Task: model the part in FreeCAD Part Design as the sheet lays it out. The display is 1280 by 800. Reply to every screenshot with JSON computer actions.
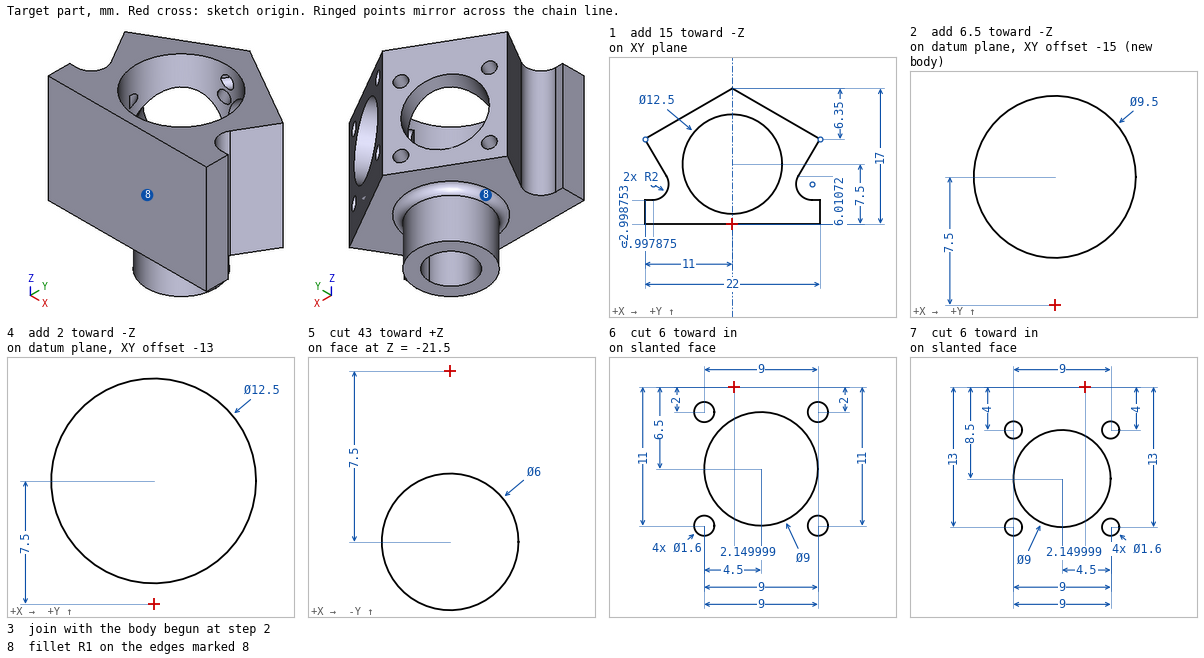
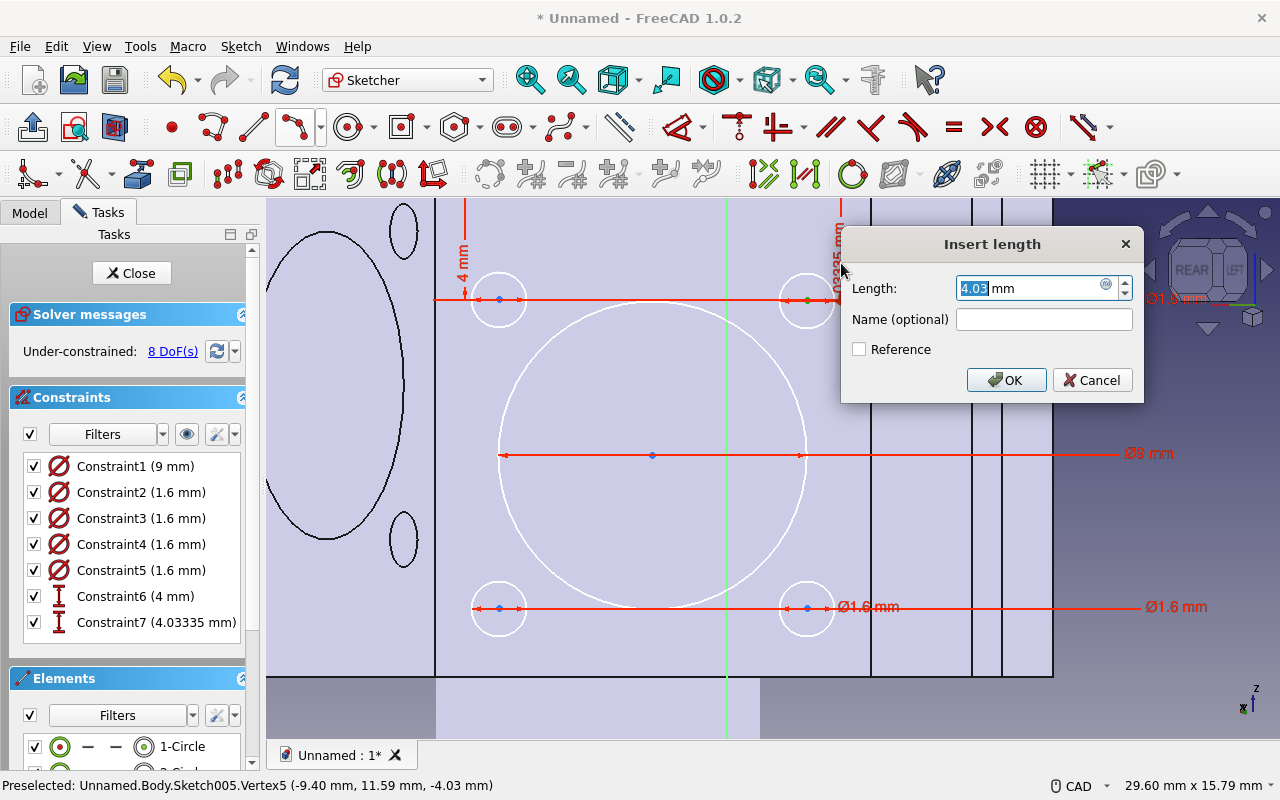
{"action": "type", "text": "4"}
{"action": "key", "text": "Return"}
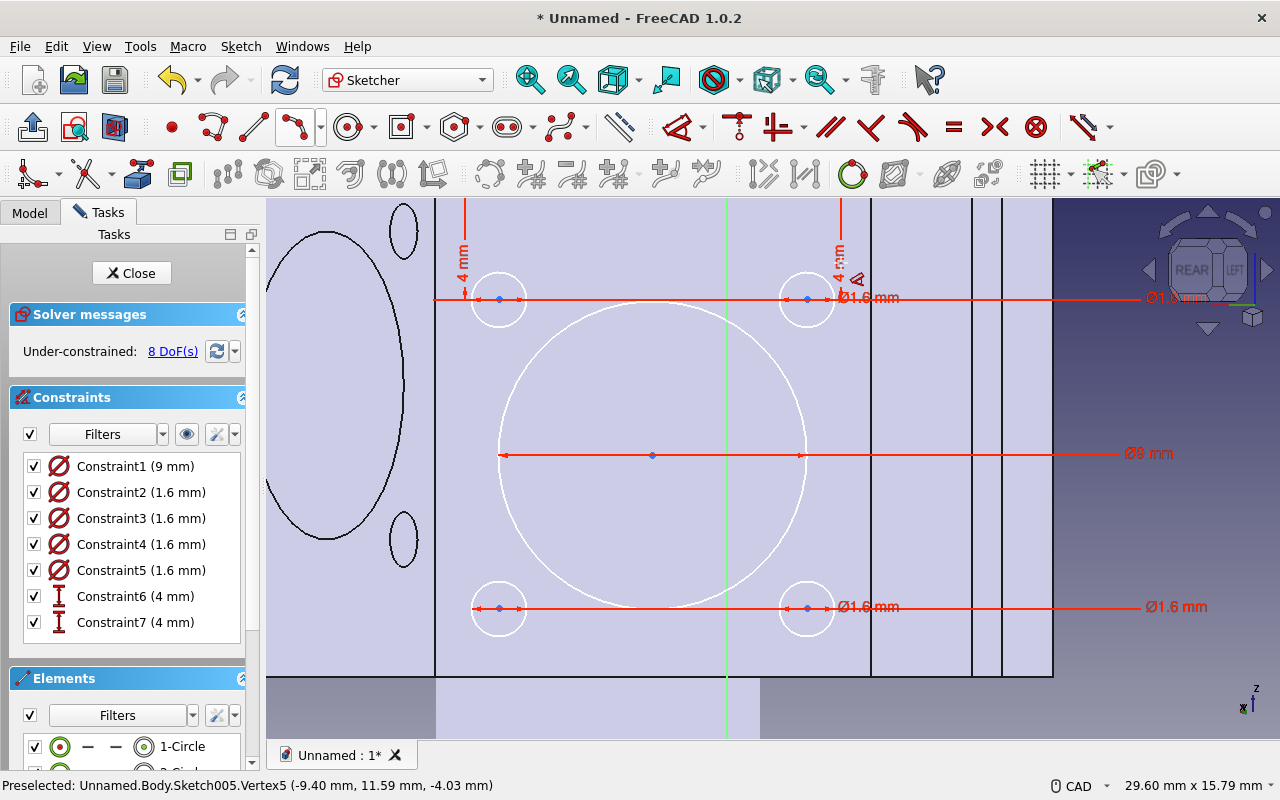
{"action": "left_click", "coordinate": [807, 609]}
{"action": "left_click", "coordinate": [841, 417]}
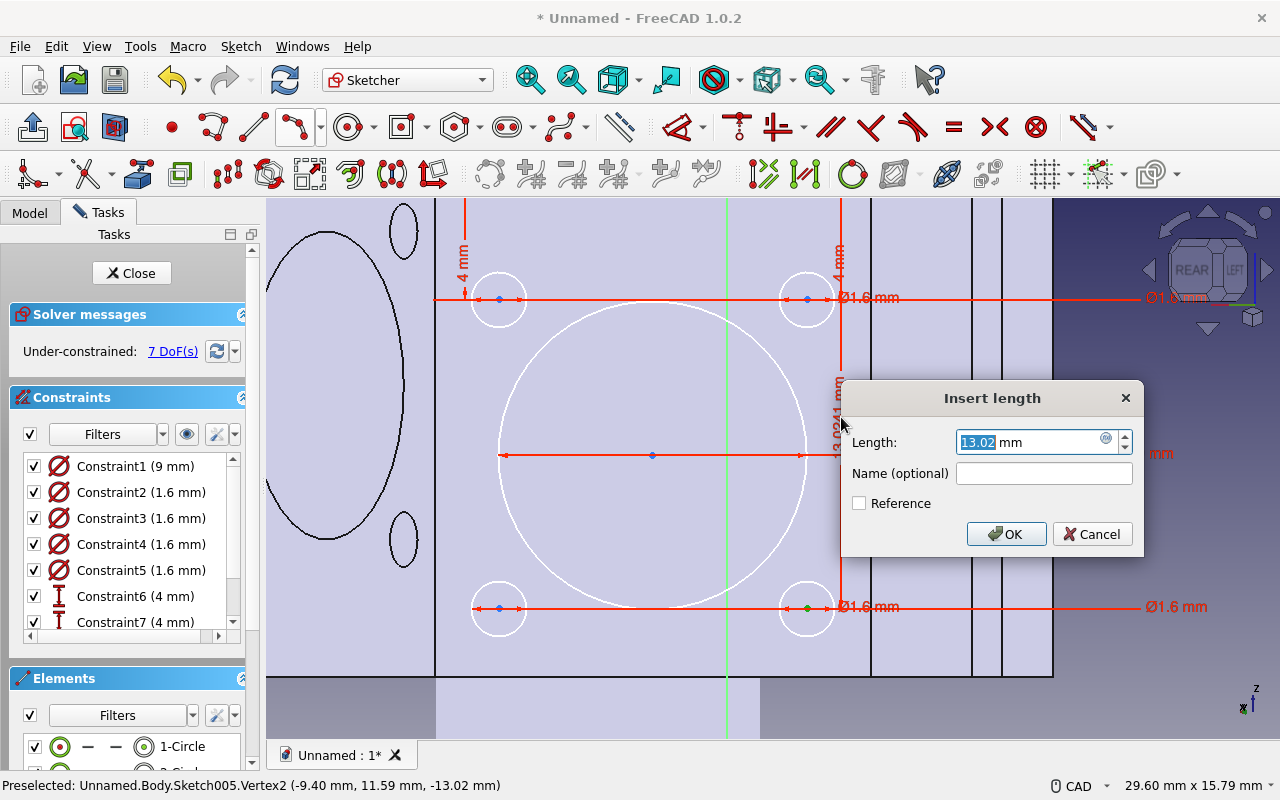
{"action": "type", "text": "13"}
{"action": "key", "text": "Return"}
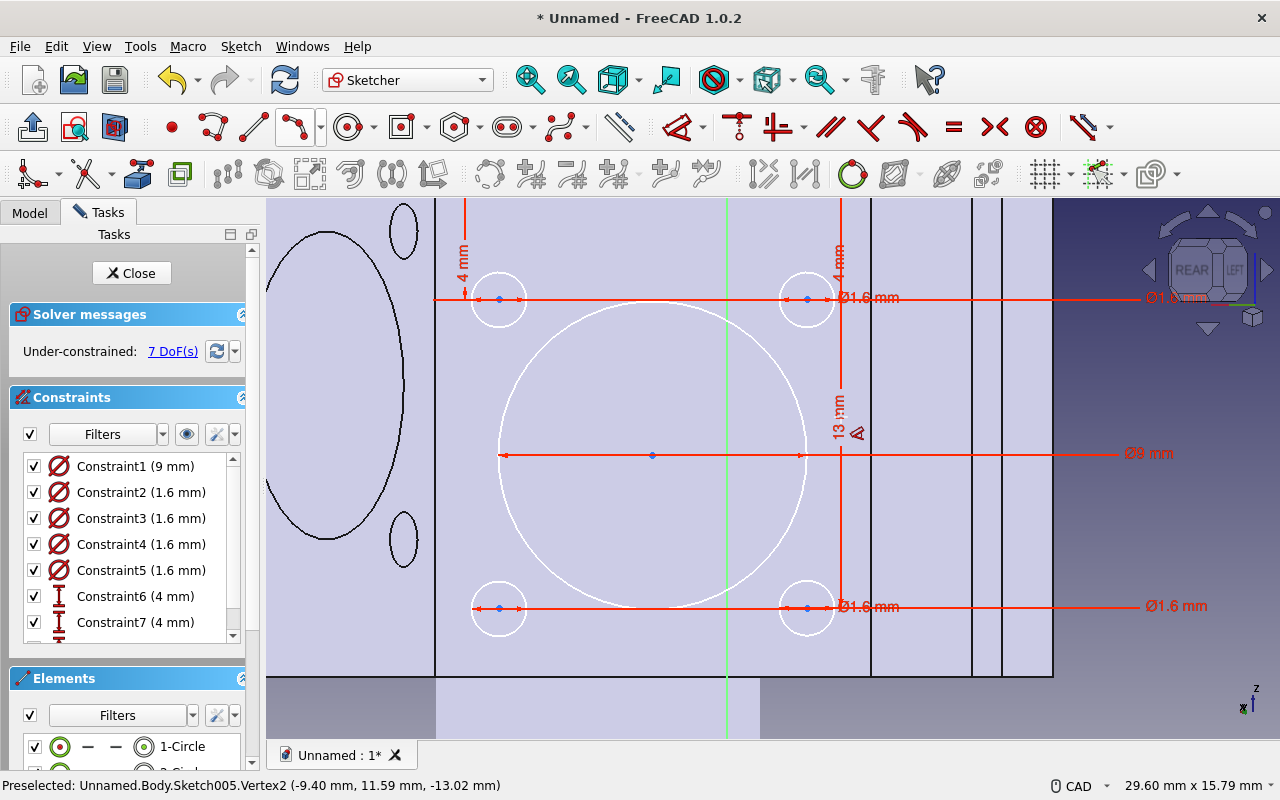
{"action": "left_click", "coordinate": [499, 609]}
{"action": "left_click", "coordinate": [465, 417]}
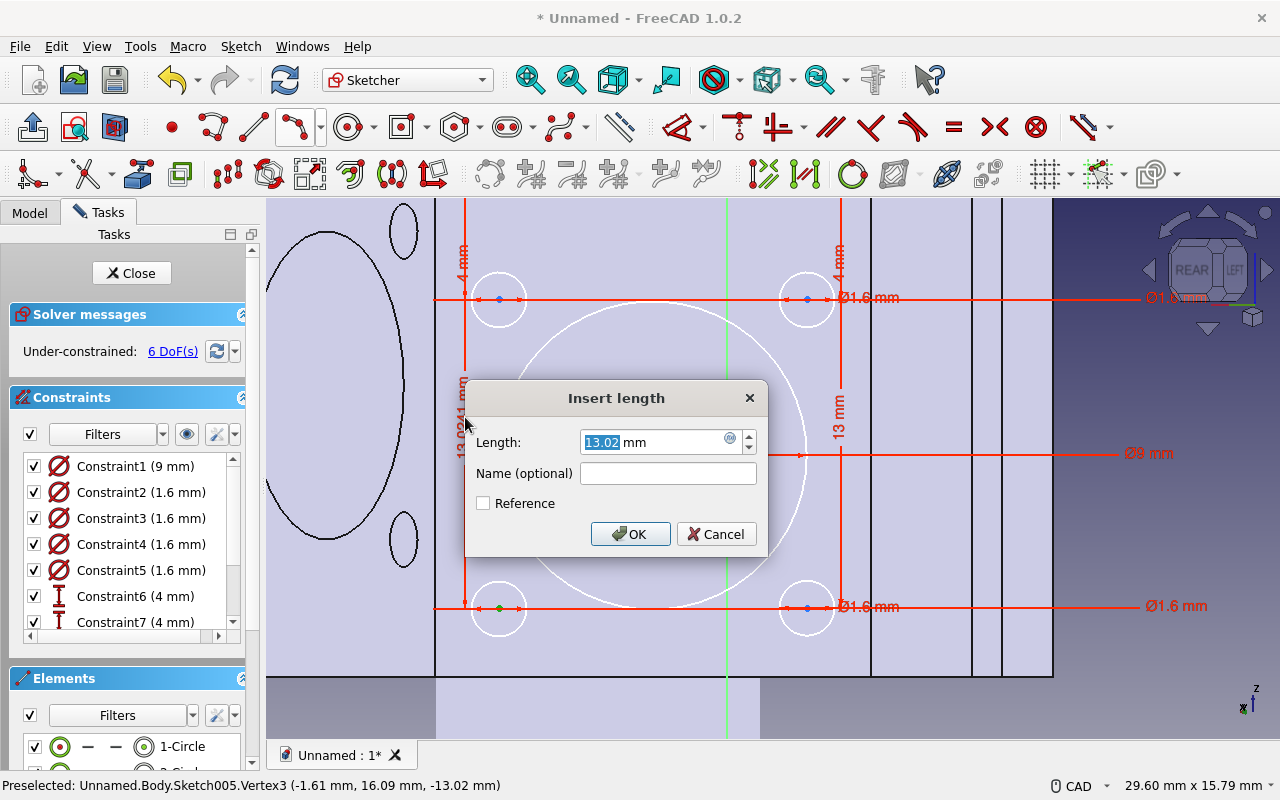
{"action": "type", "text": "13"}
{"action": "key", "text": "Return"}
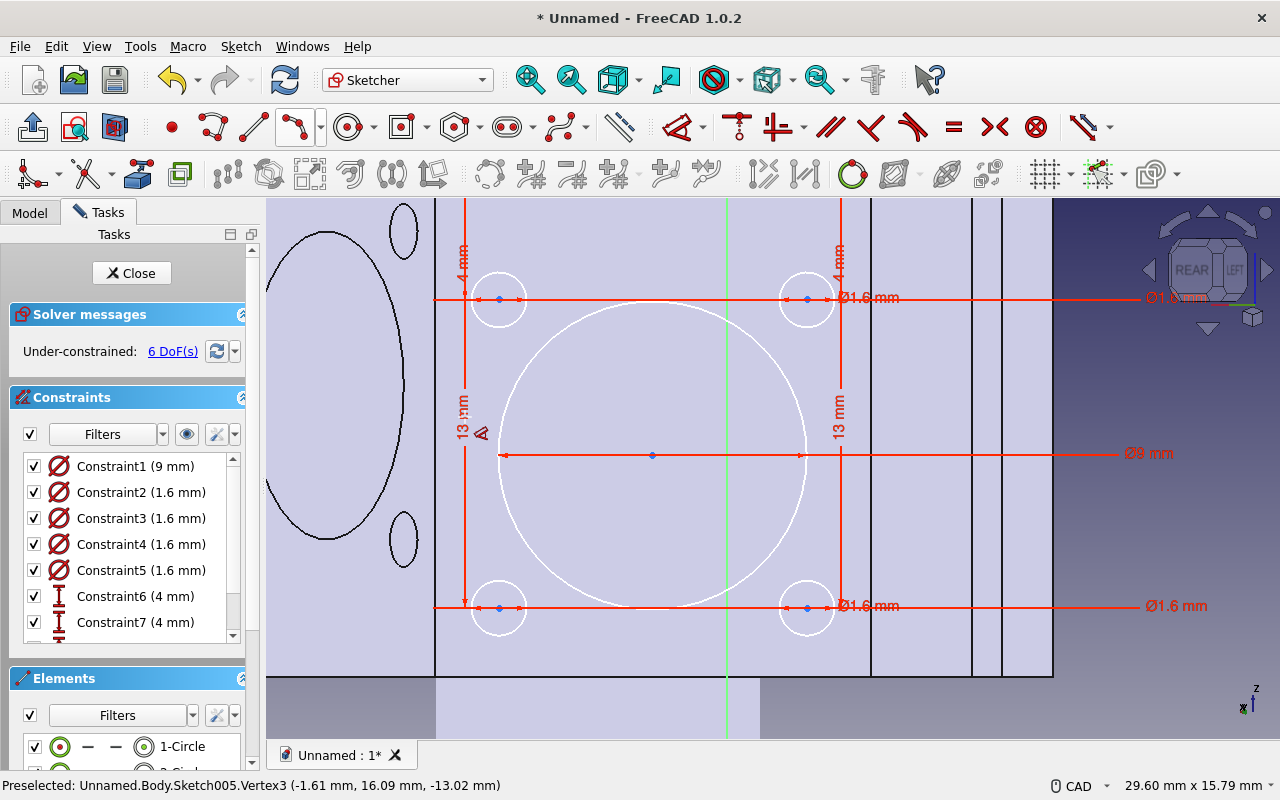
{"action": "left_click", "coordinate": [807, 608]}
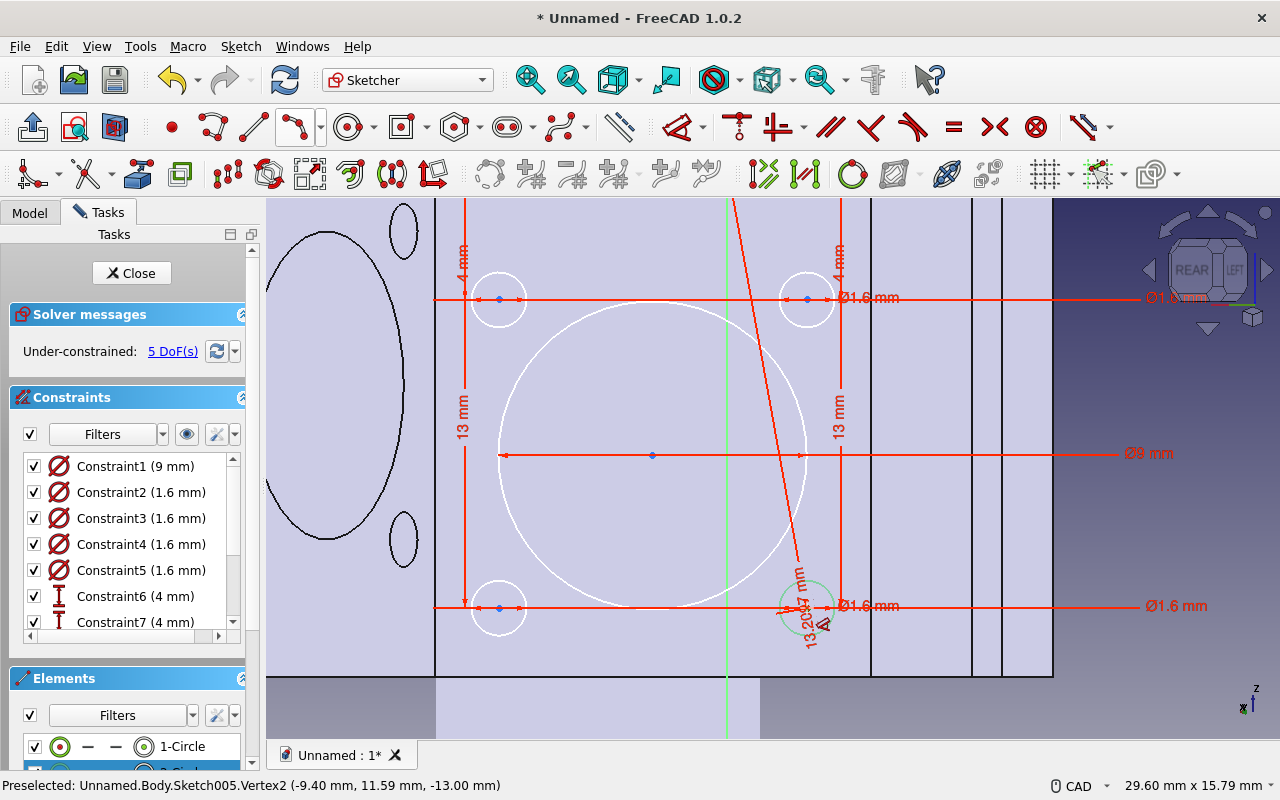
{"action": "left_click", "coordinate": [499, 608]}
{"action": "left_click", "coordinate": [653, 642]}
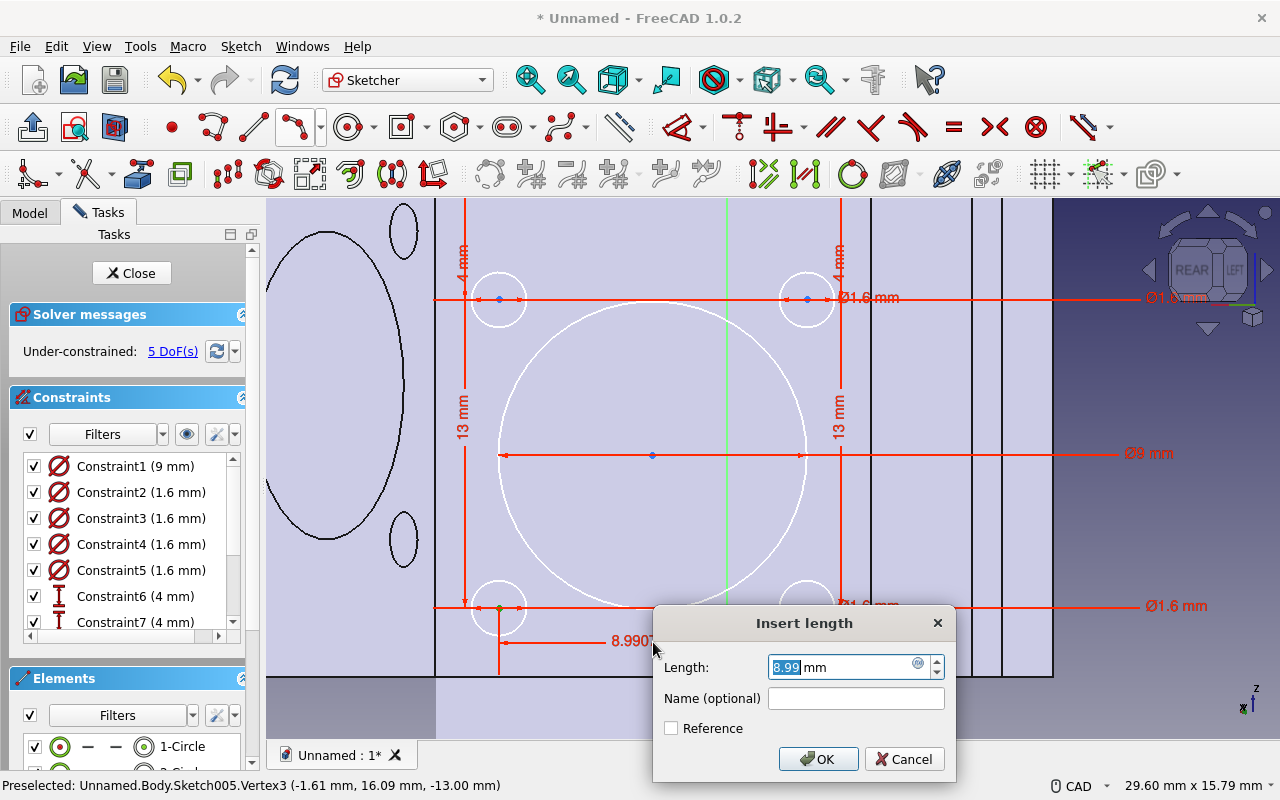
{"action": "type", "text": "9"}
{"action": "key", "text": "Return"}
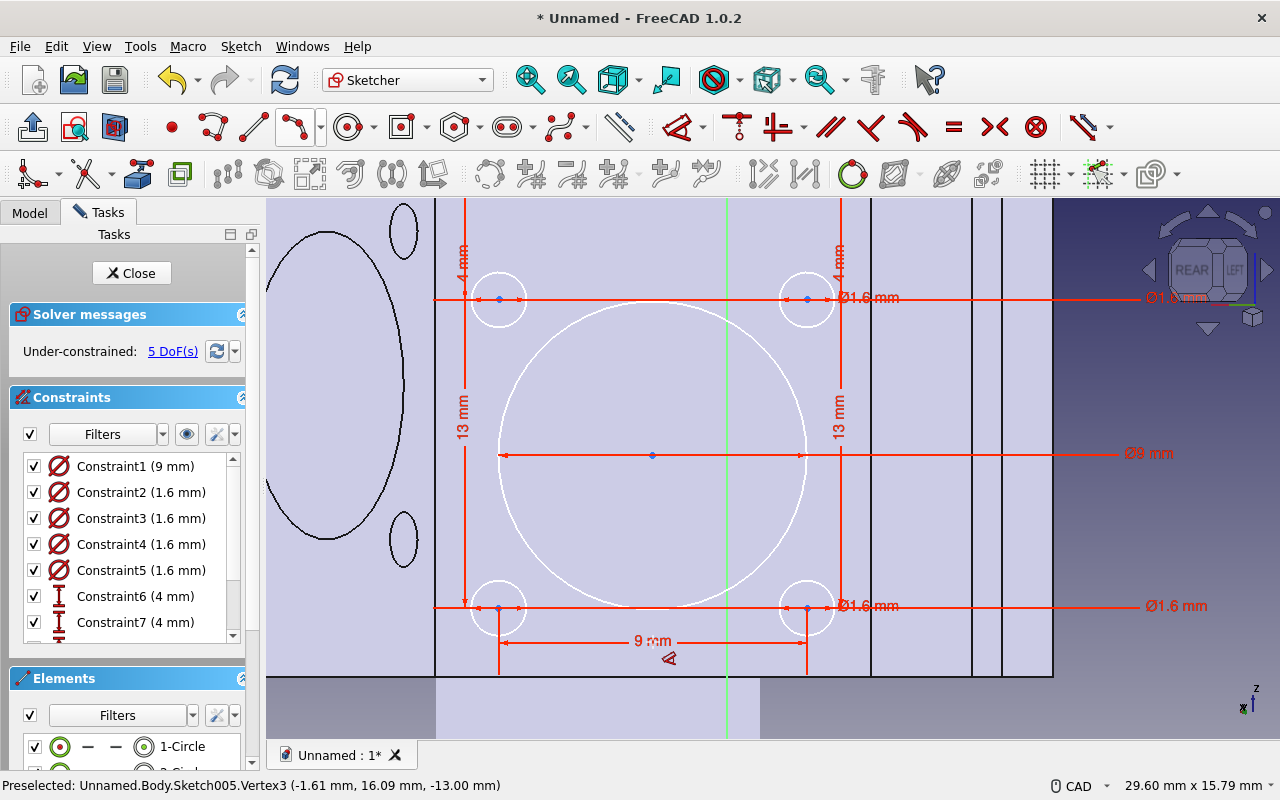
{"action": "left_click", "coordinate": [807, 608]}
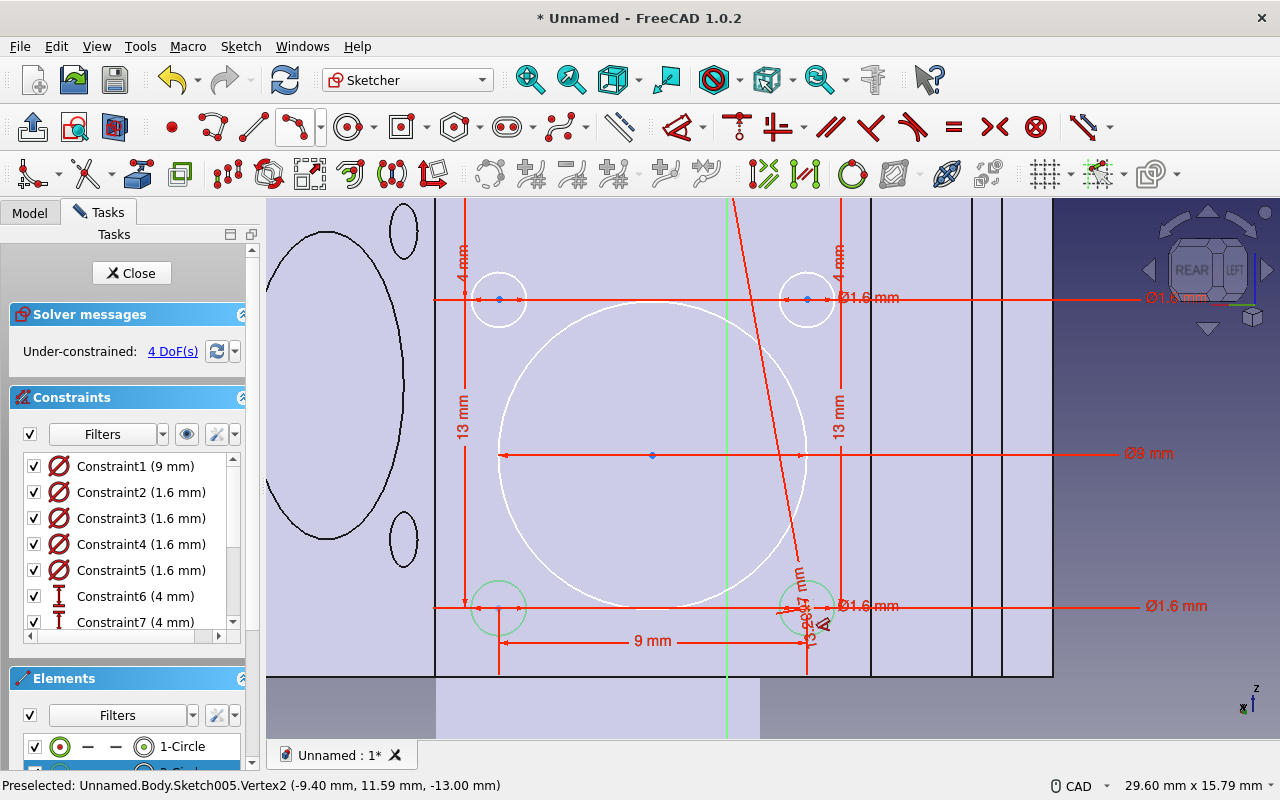
{"action": "left_click", "coordinate": [499, 300]}
{"action": "left_click", "coordinate": [582, 642]}